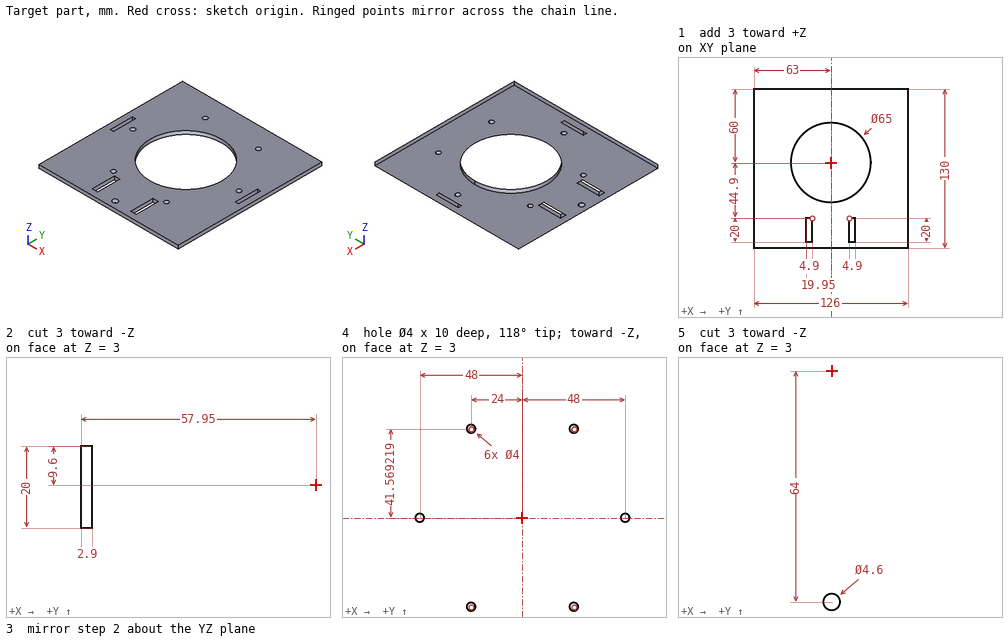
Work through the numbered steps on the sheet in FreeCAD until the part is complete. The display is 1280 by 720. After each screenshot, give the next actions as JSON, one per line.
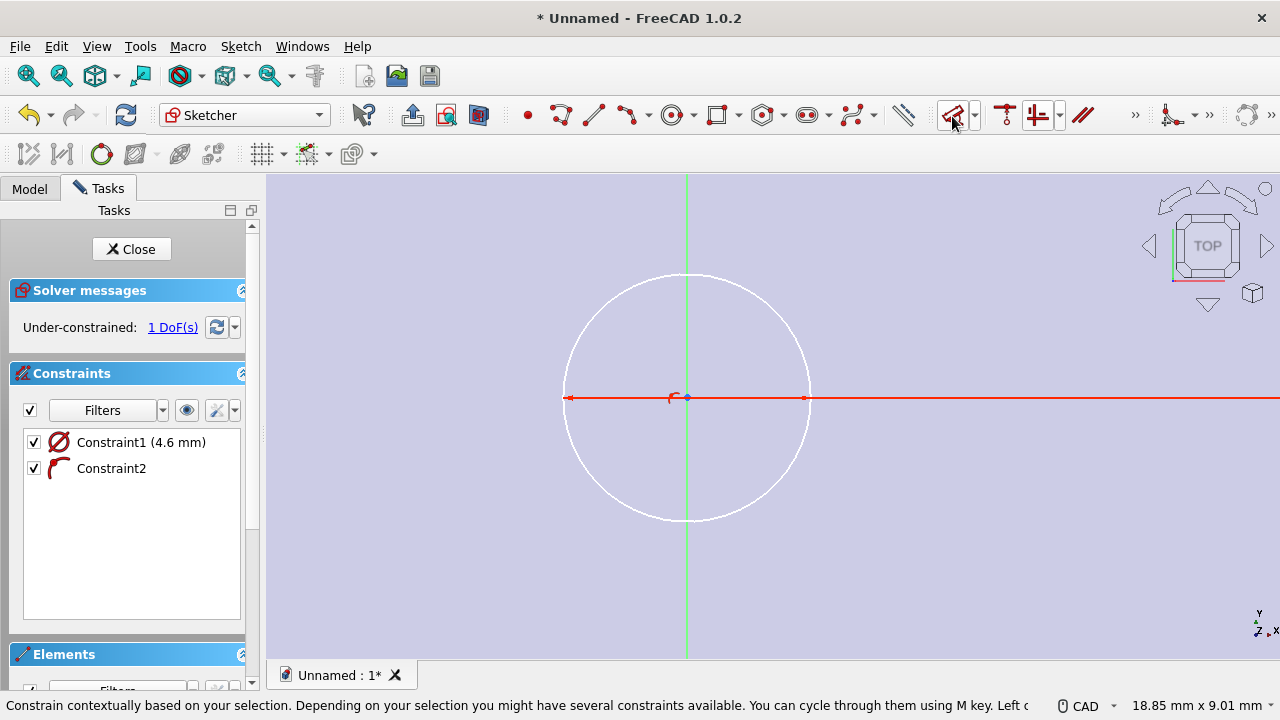
{"action": "left_click", "coordinate": [687, 398]}
{"action": "left_click", "coordinate": [721, 300]}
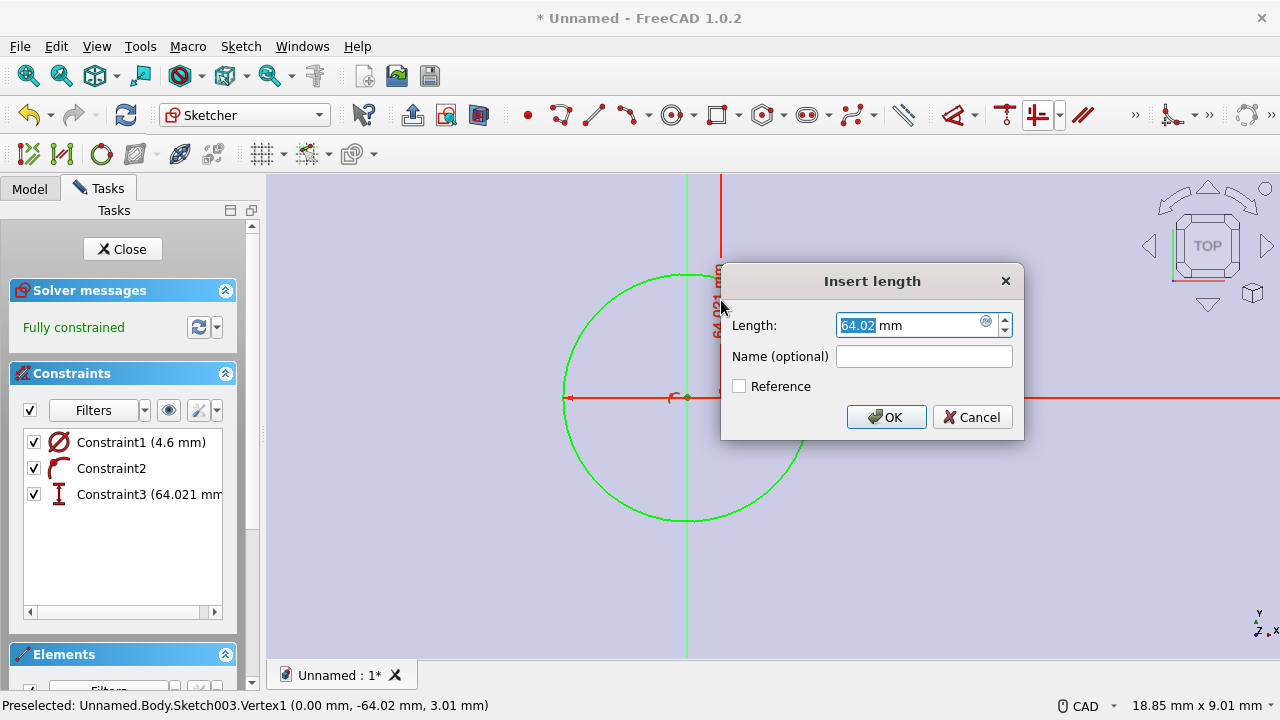
{"action": "type", "text": "64"}
{"action": "key", "text": "Return"}
{"action": "key", "text": "Escape"}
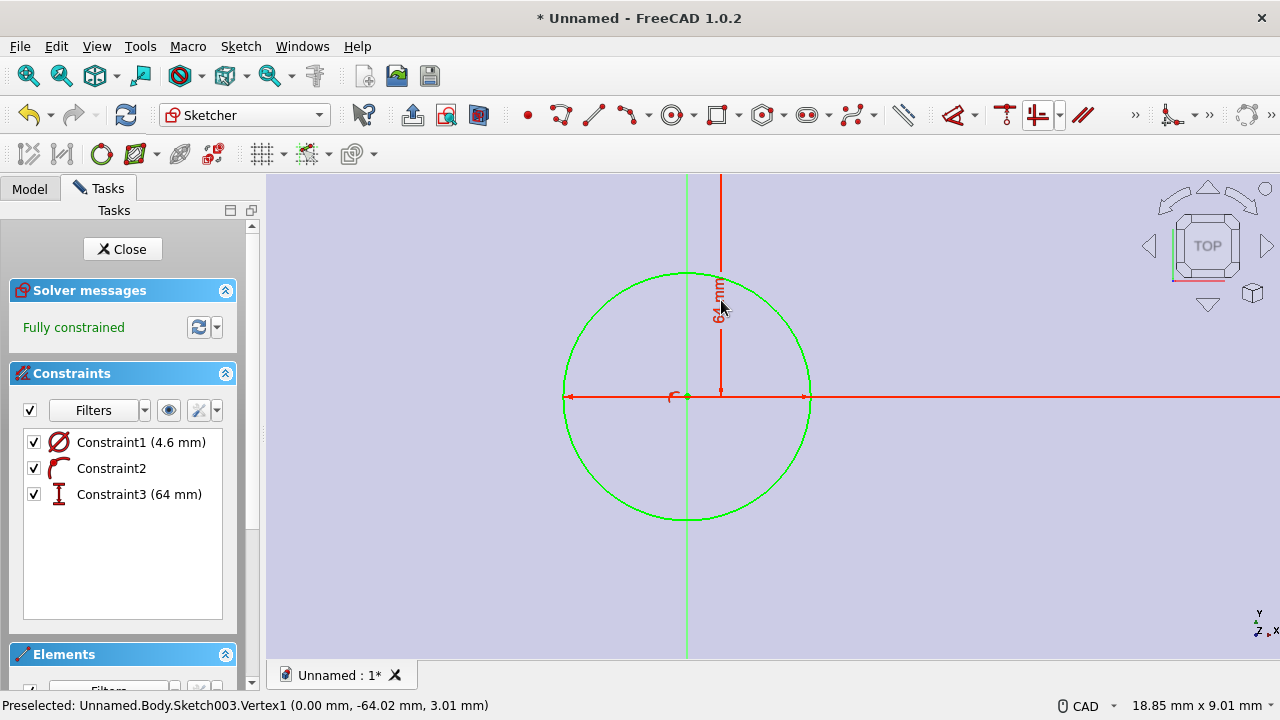
{"action": "left_click", "coordinate": [123, 249]}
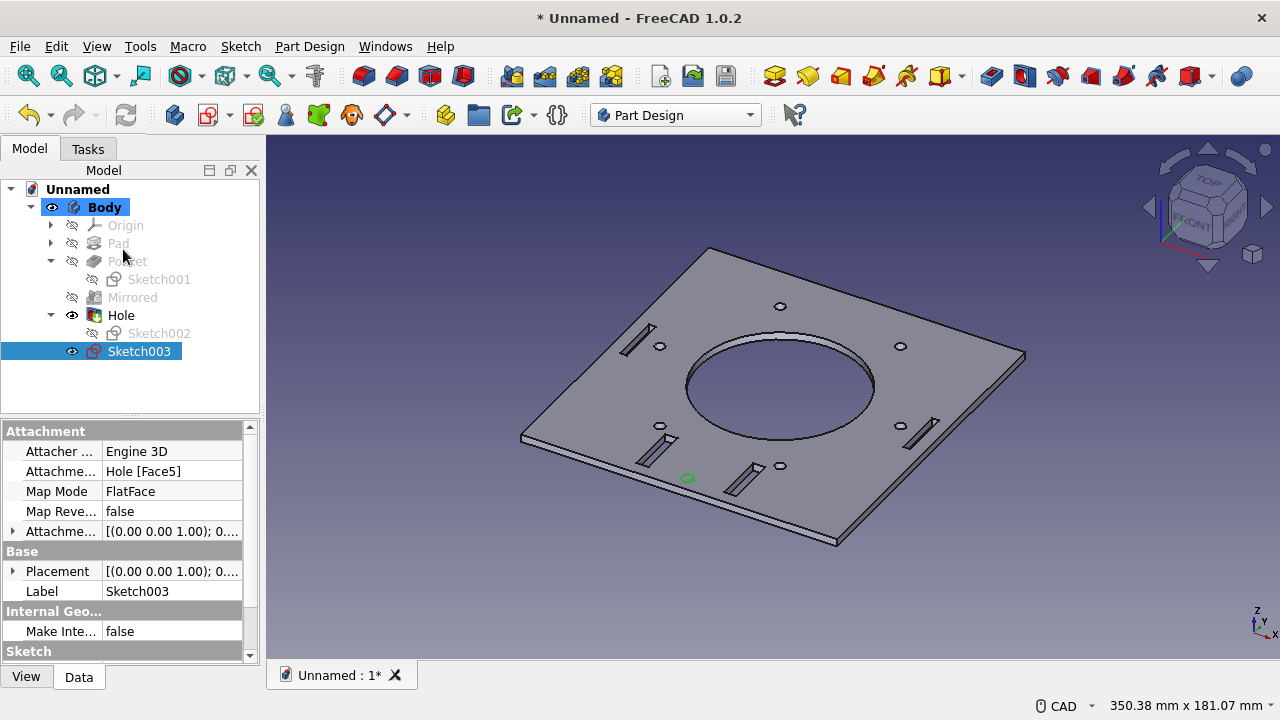
{"action": "left_click", "coordinate": [992, 76]}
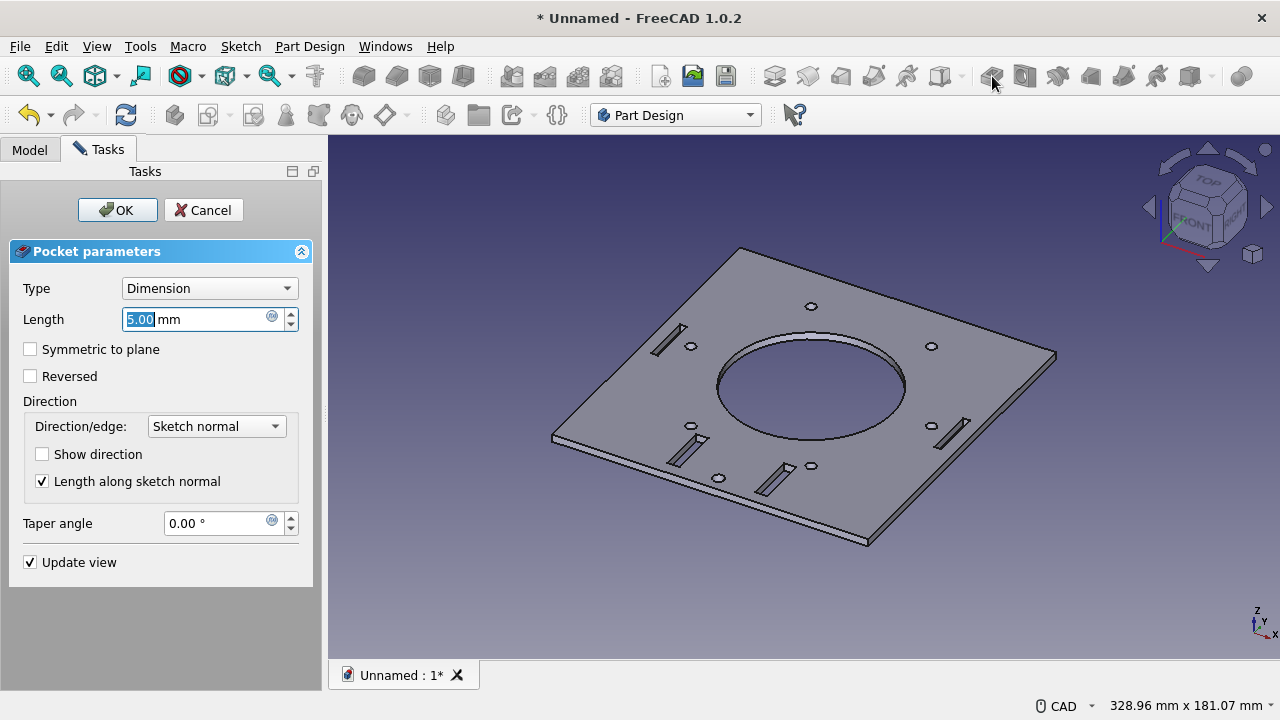
{"action": "type", "text": "3"}
{"action": "key", "text": "Tab"}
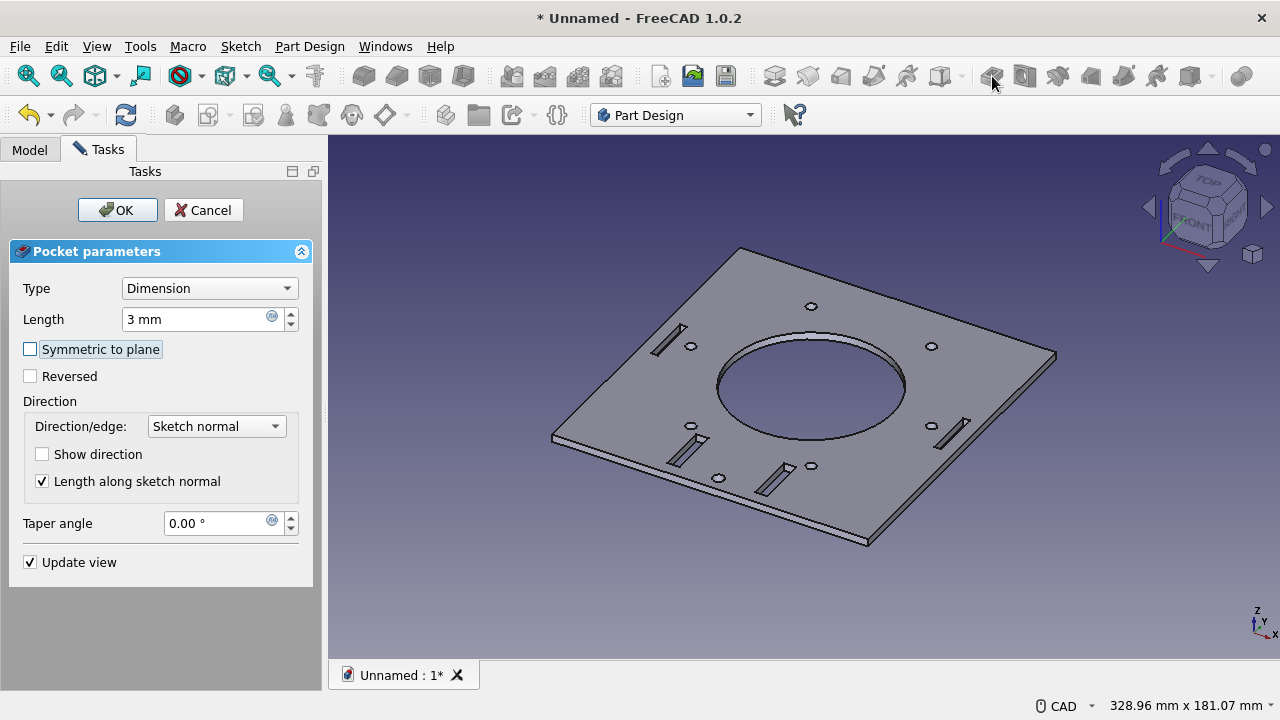
{"action": "left_click", "coordinate": [118, 210]}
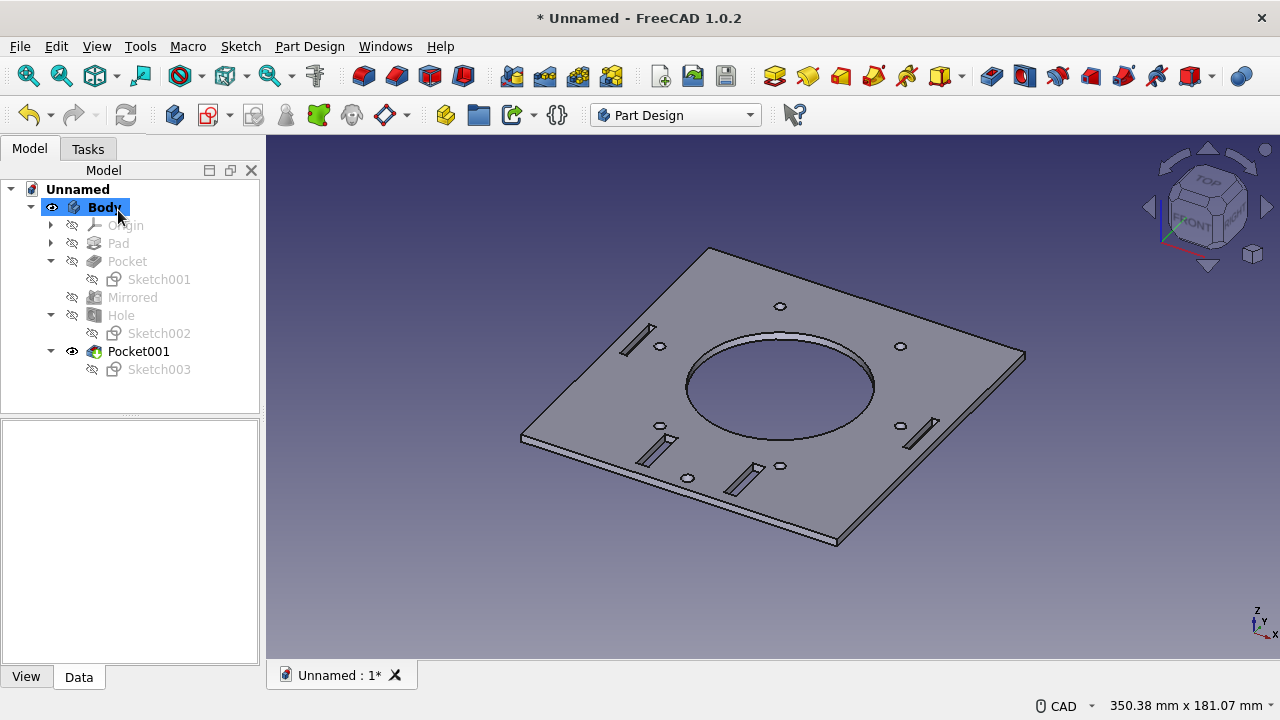
{"action": "key", "text": "0"}